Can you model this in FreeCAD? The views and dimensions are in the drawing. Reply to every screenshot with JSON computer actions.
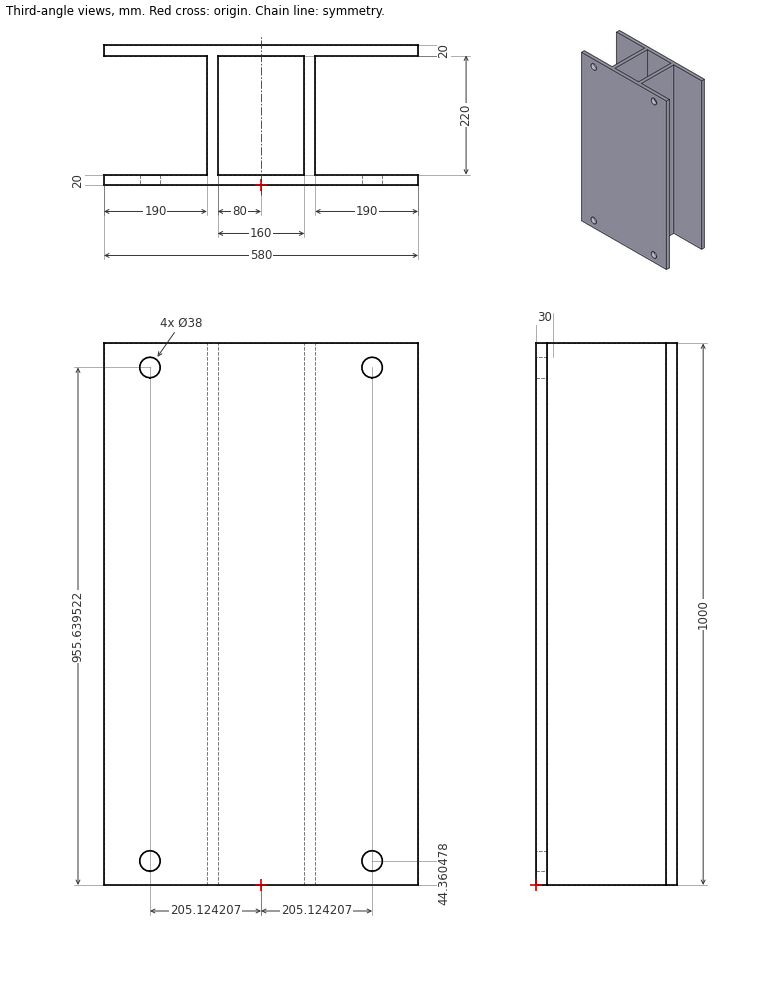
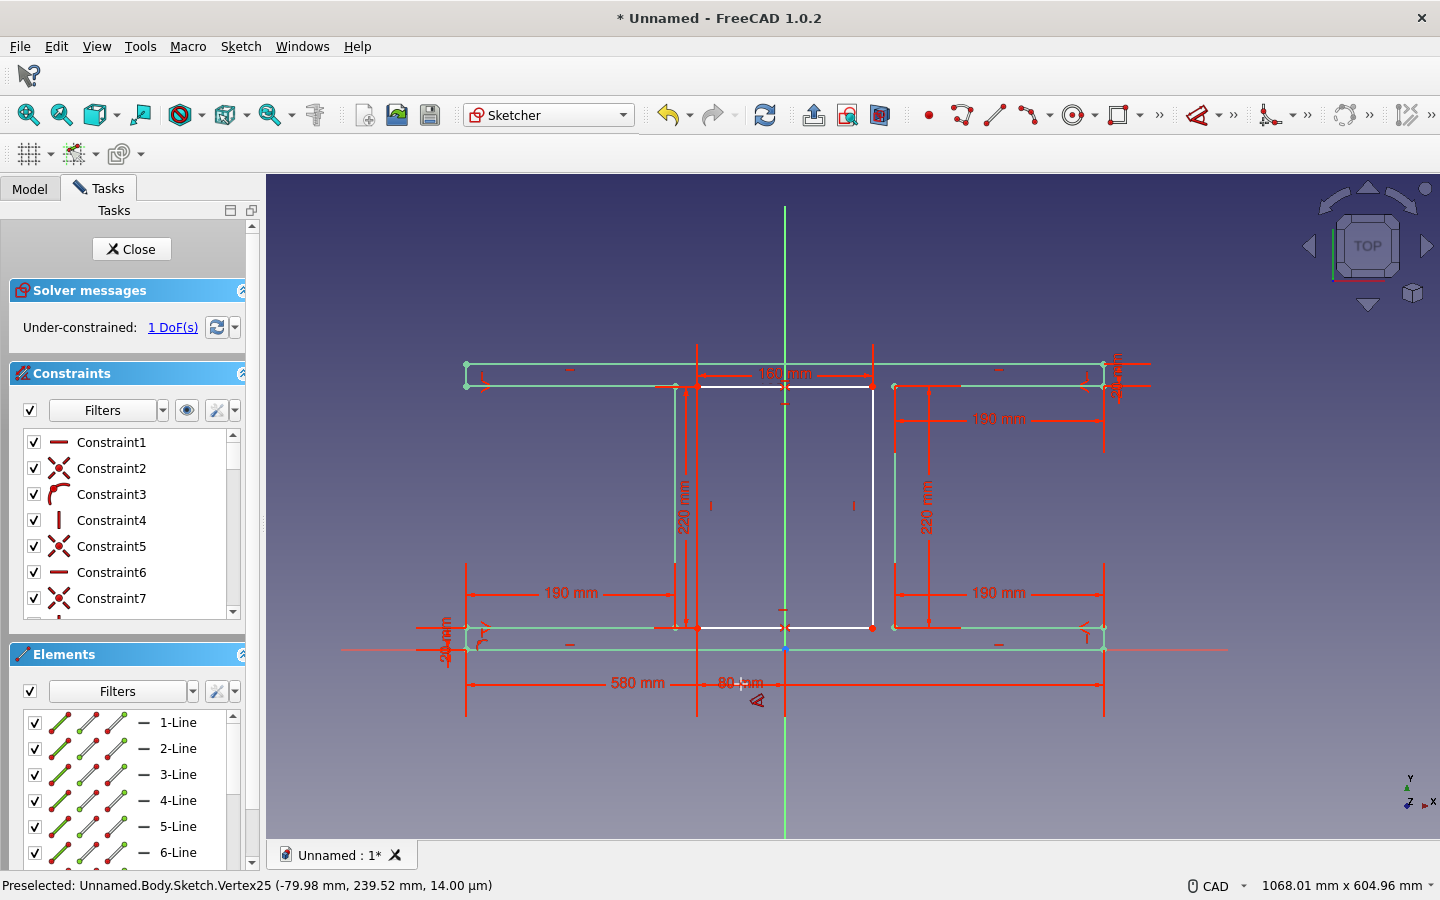
{"action": "scroll", "coordinate": [697, 628], "scroll_direction": "up", "scroll_amount": 3}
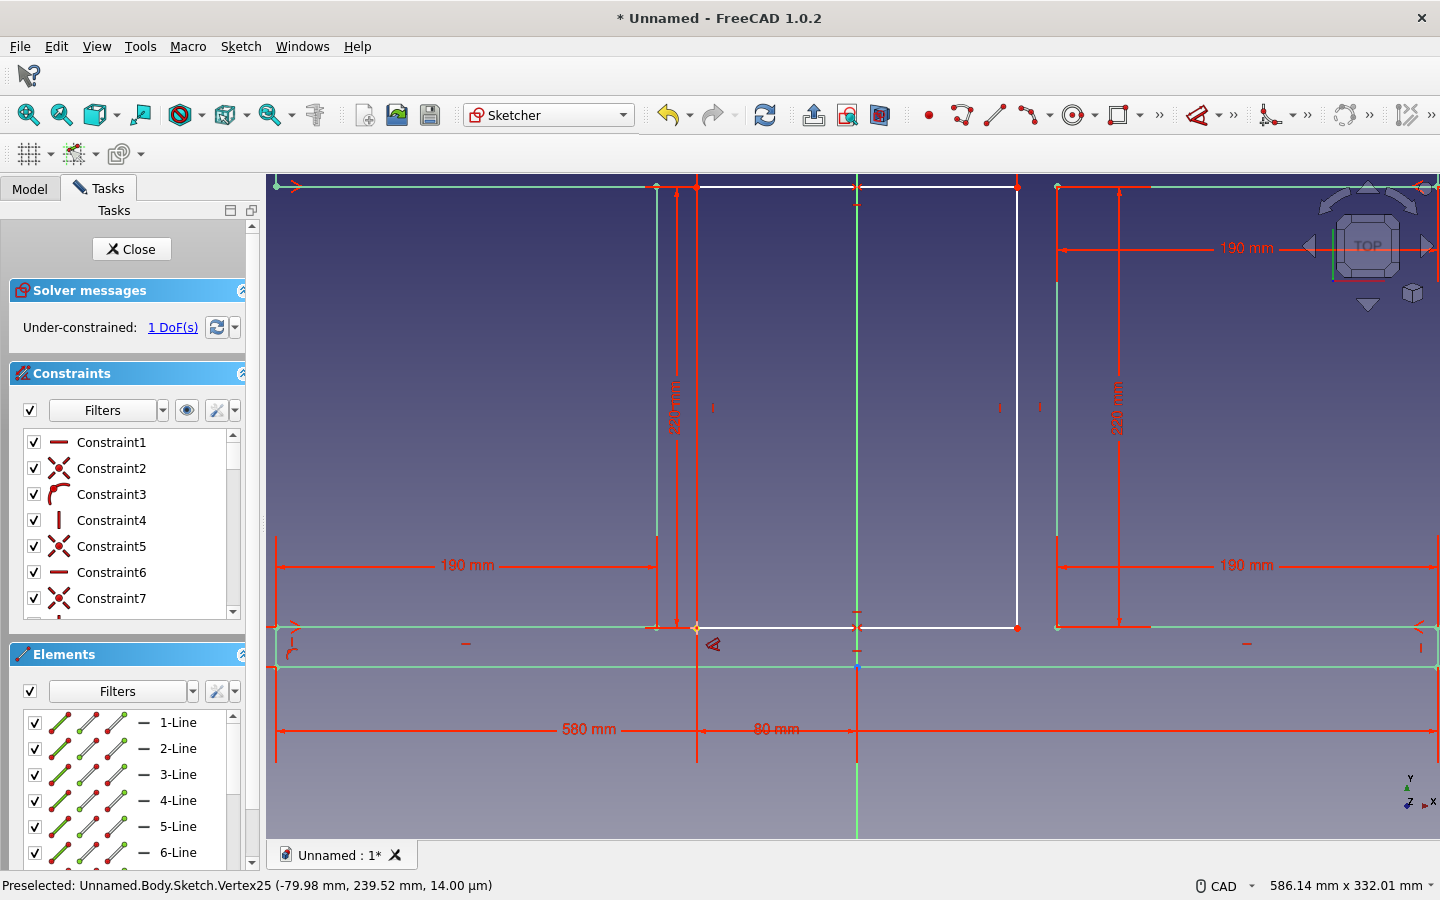
{"action": "left_click", "coordinate": [697, 628]}
{"action": "left_click", "coordinate": [663, 648]}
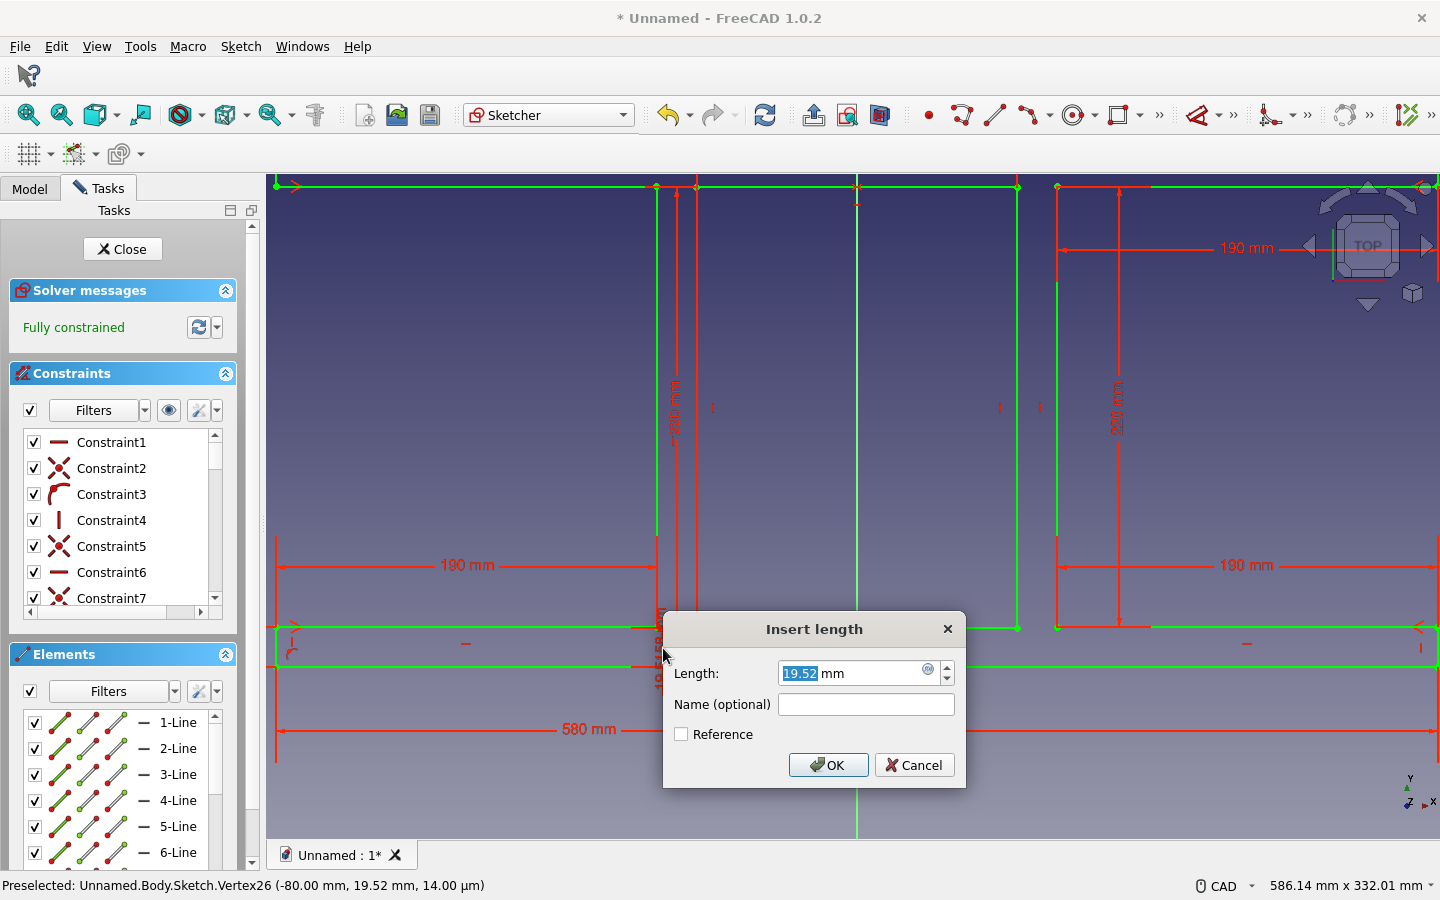
{"action": "type", "text": "20"}
{"action": "key", "text": "Return"}
{"action": "key", "text": "Escape"}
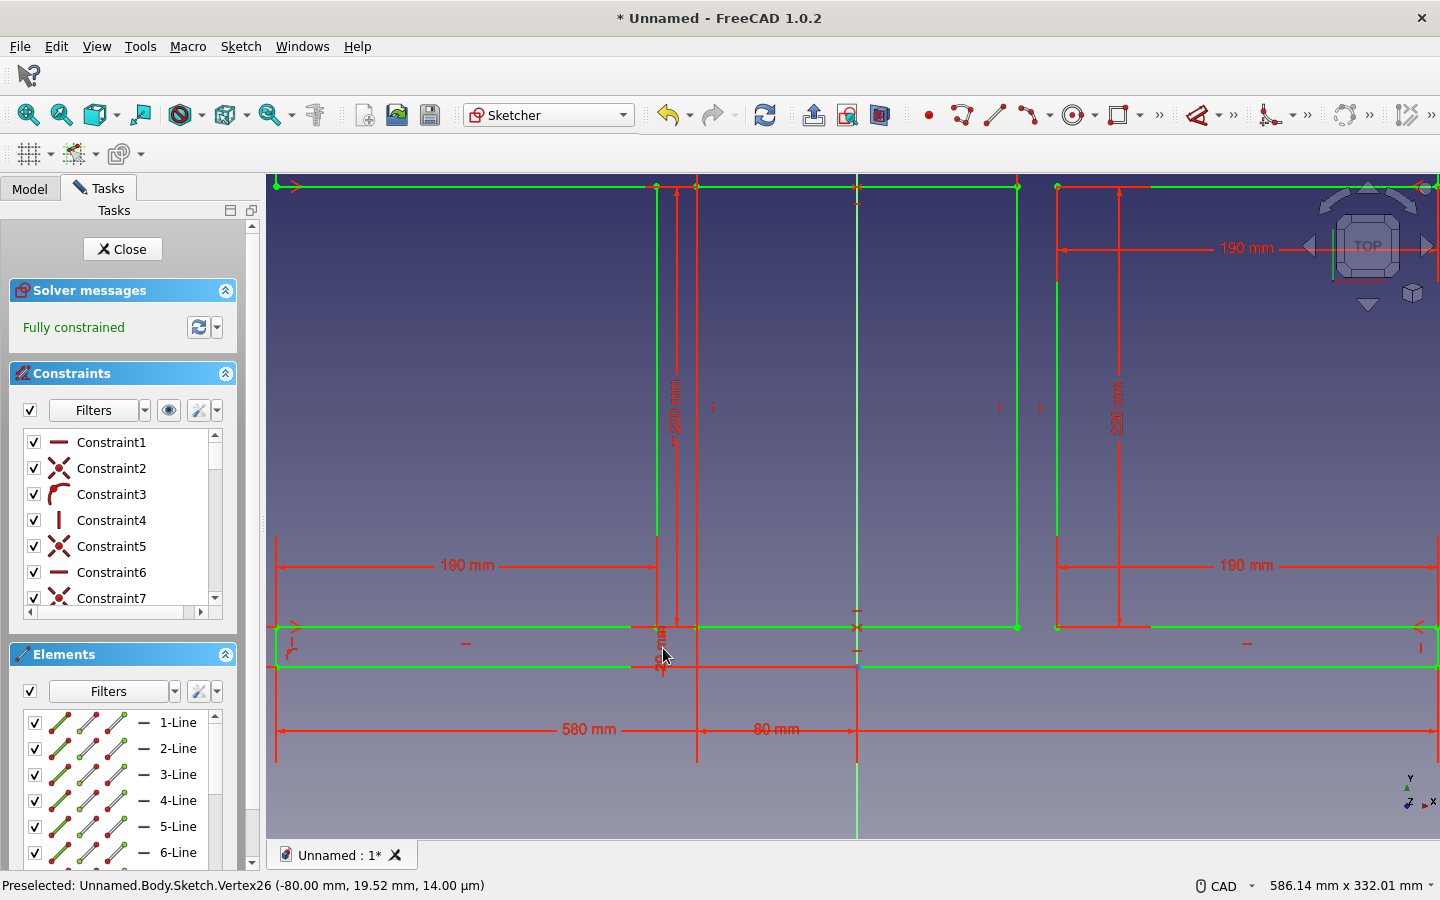
{"action": "left_click", "coordinate": [123, 249]}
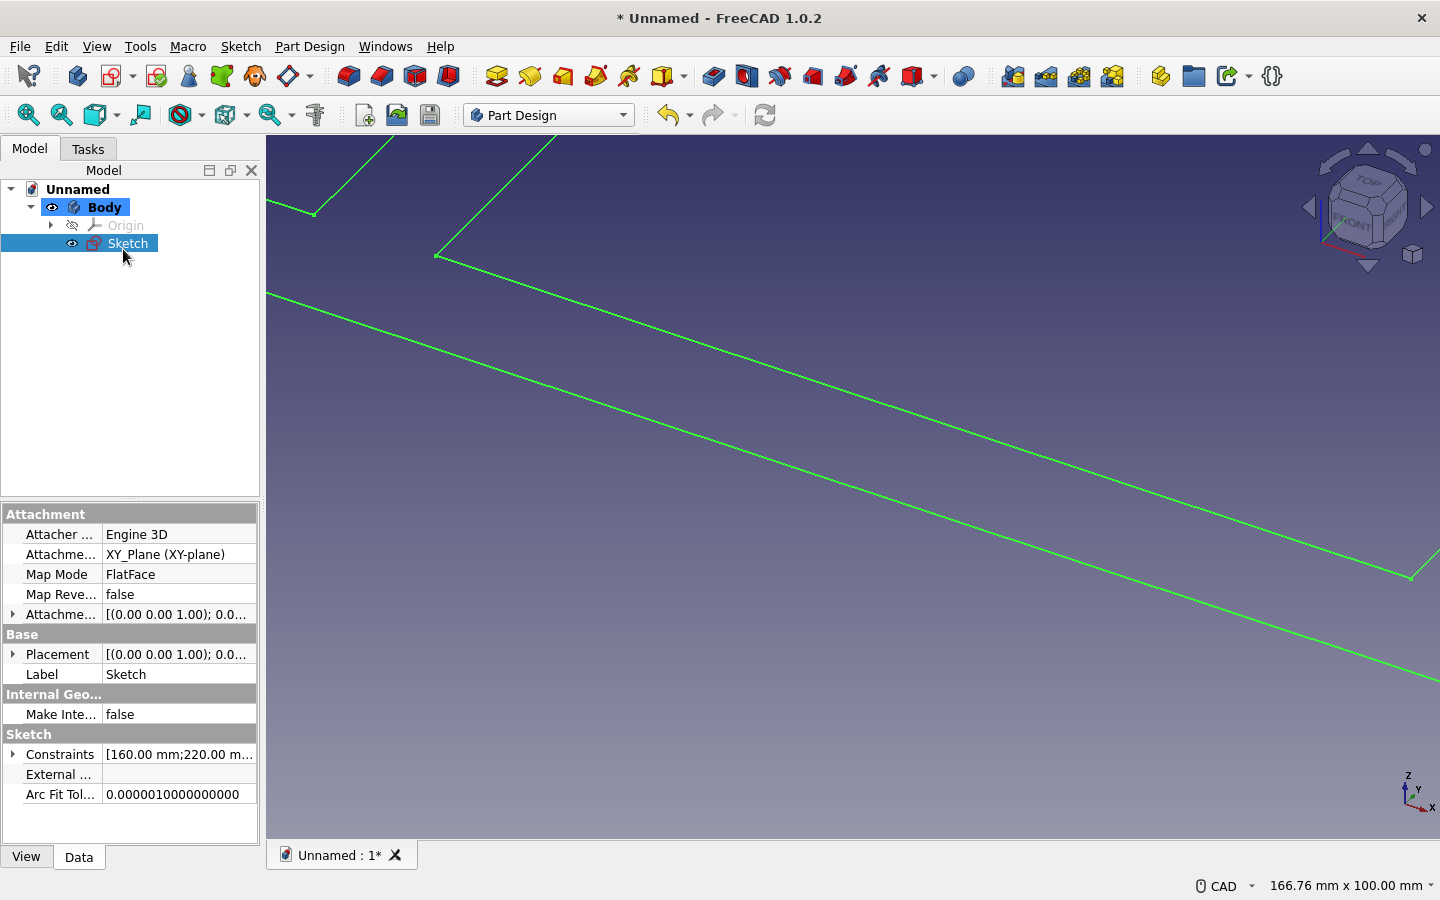
{"action": "left_click", "coordinate": [497, 76]}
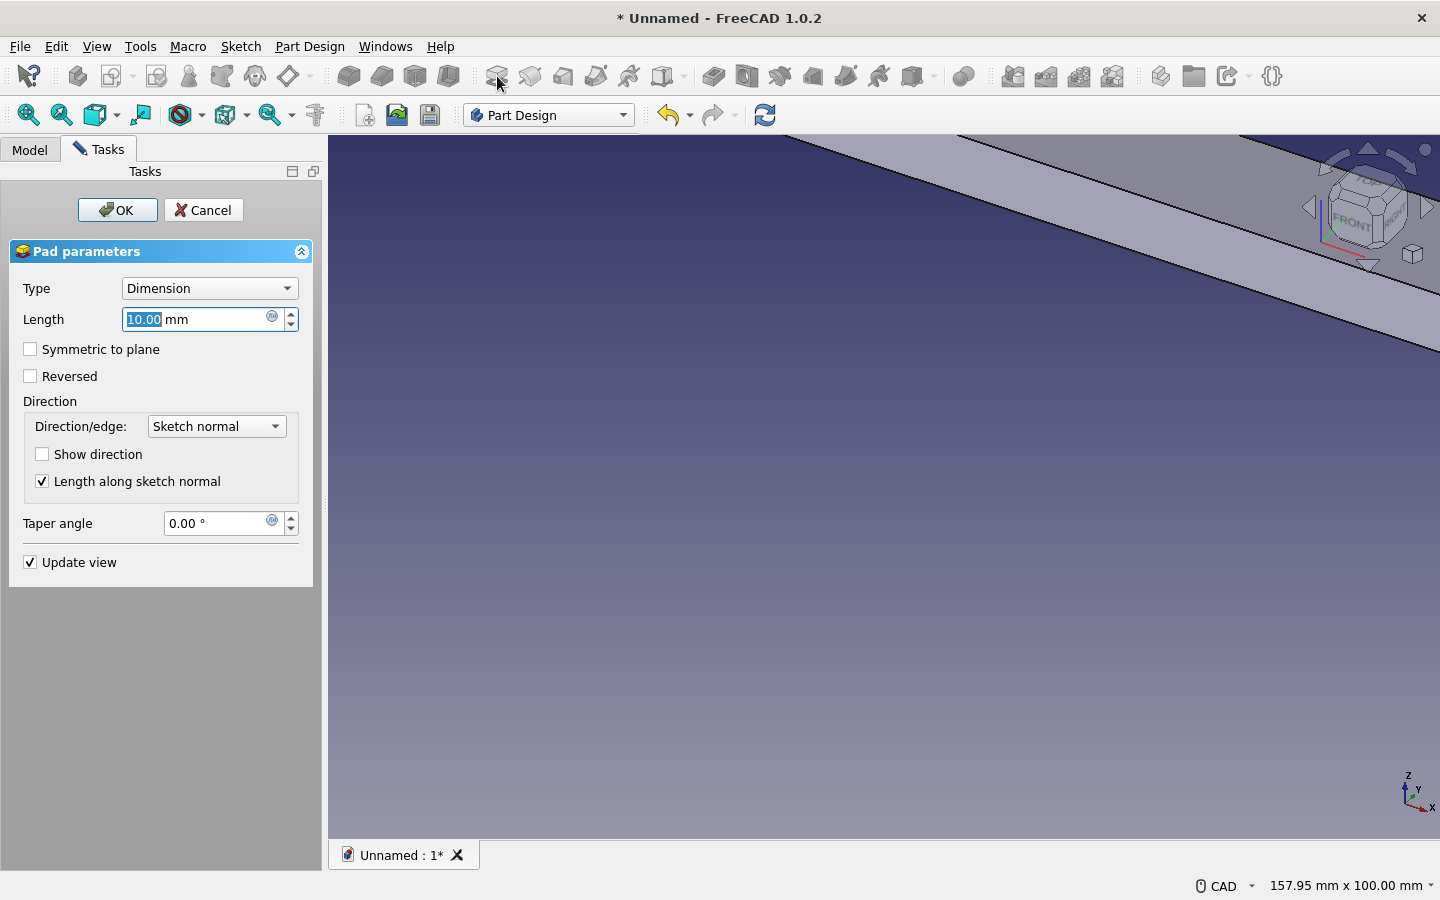
{"action": "type", "text": "1000"}
{"action": "key", "text": "Tab"}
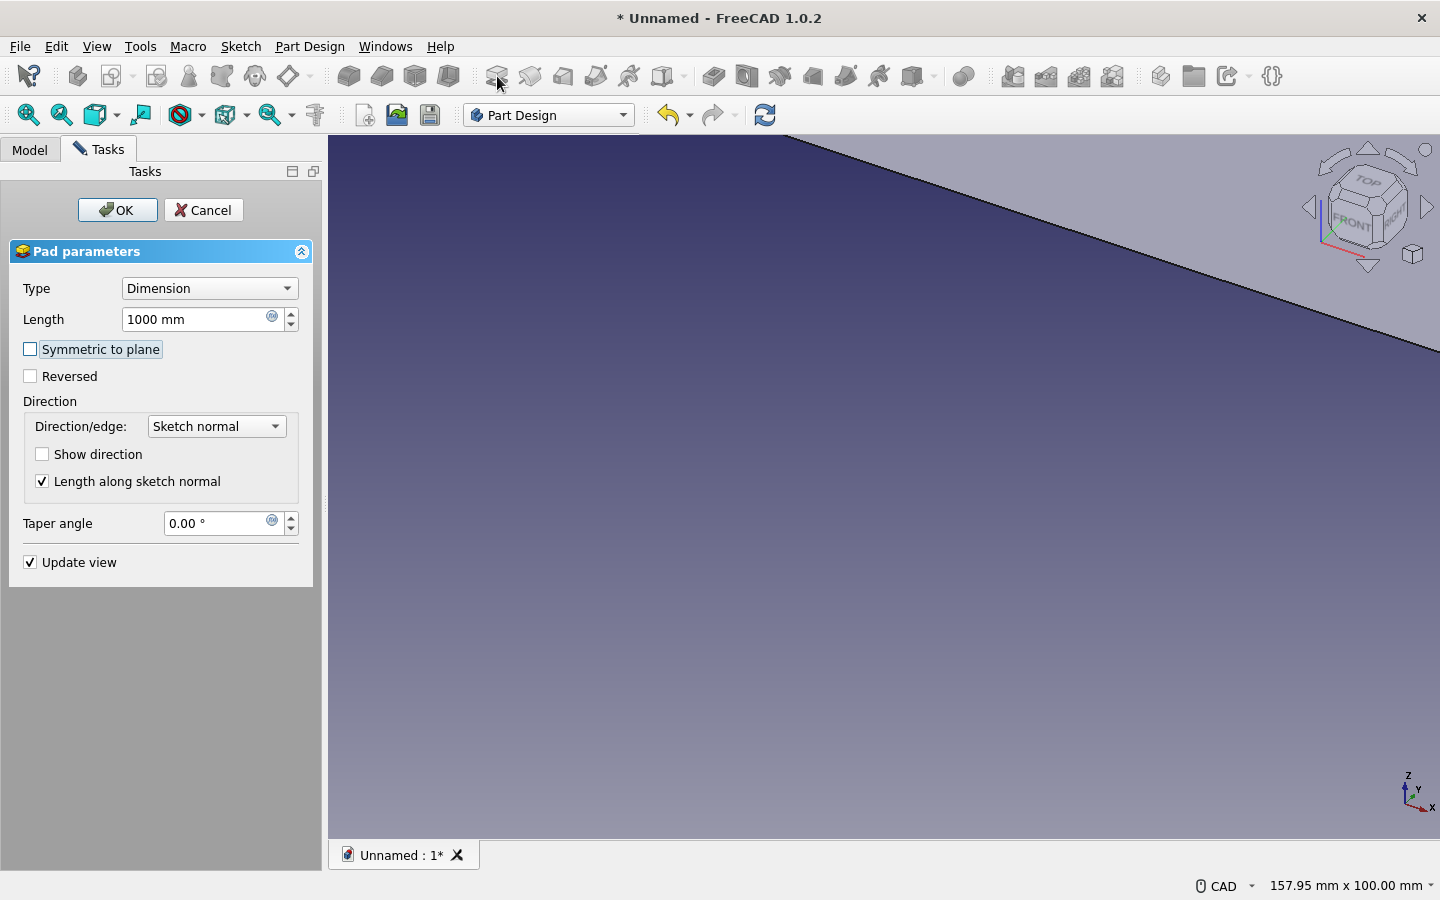
{"action": "left_click", "coordinate": [118, 210]}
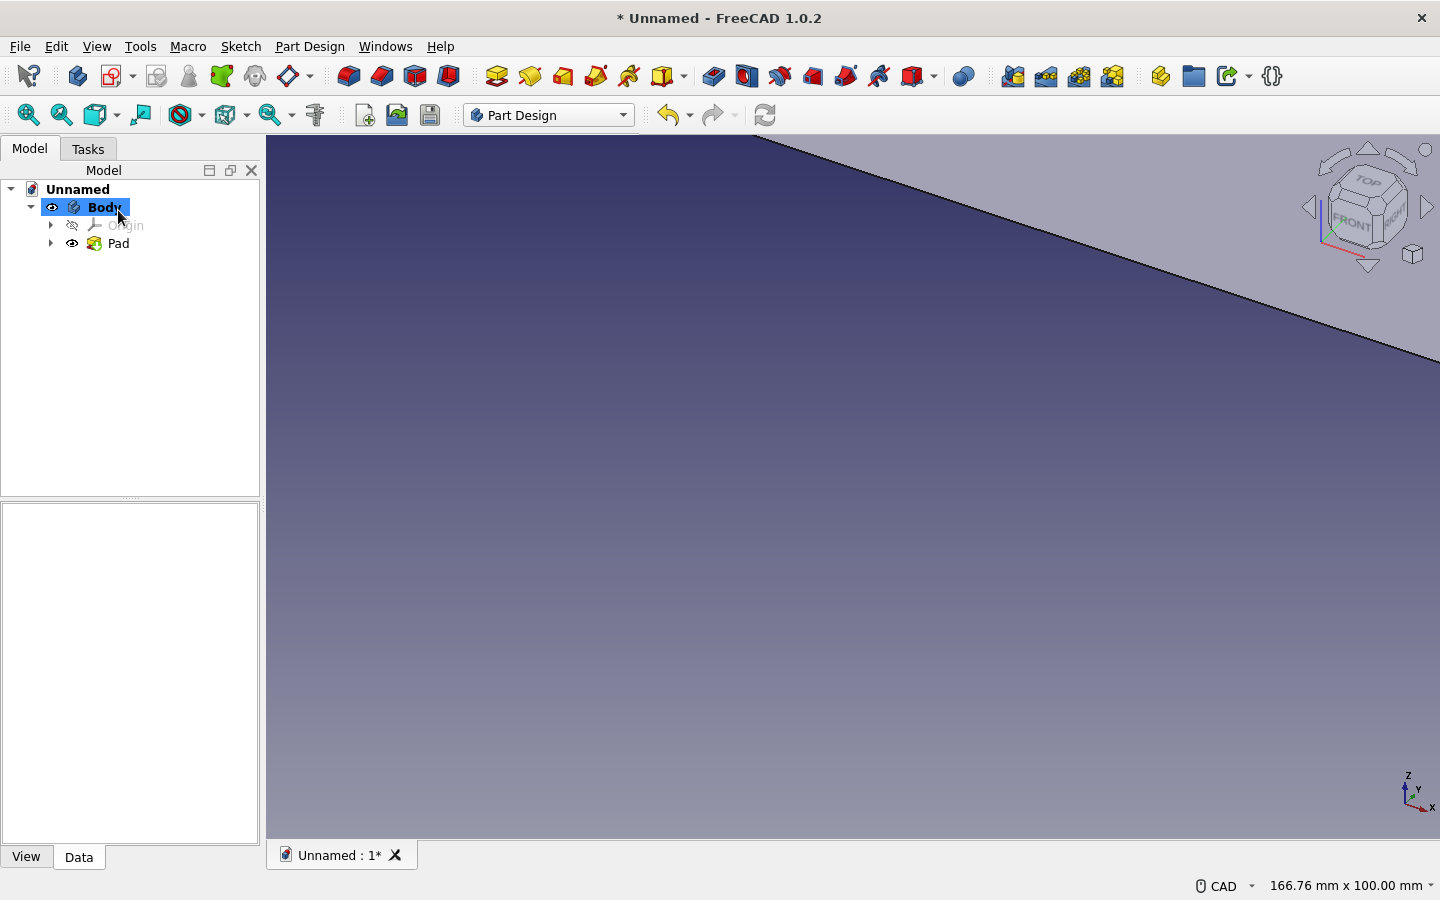
{"action": "left_click", "coordinate": [29, 116]}